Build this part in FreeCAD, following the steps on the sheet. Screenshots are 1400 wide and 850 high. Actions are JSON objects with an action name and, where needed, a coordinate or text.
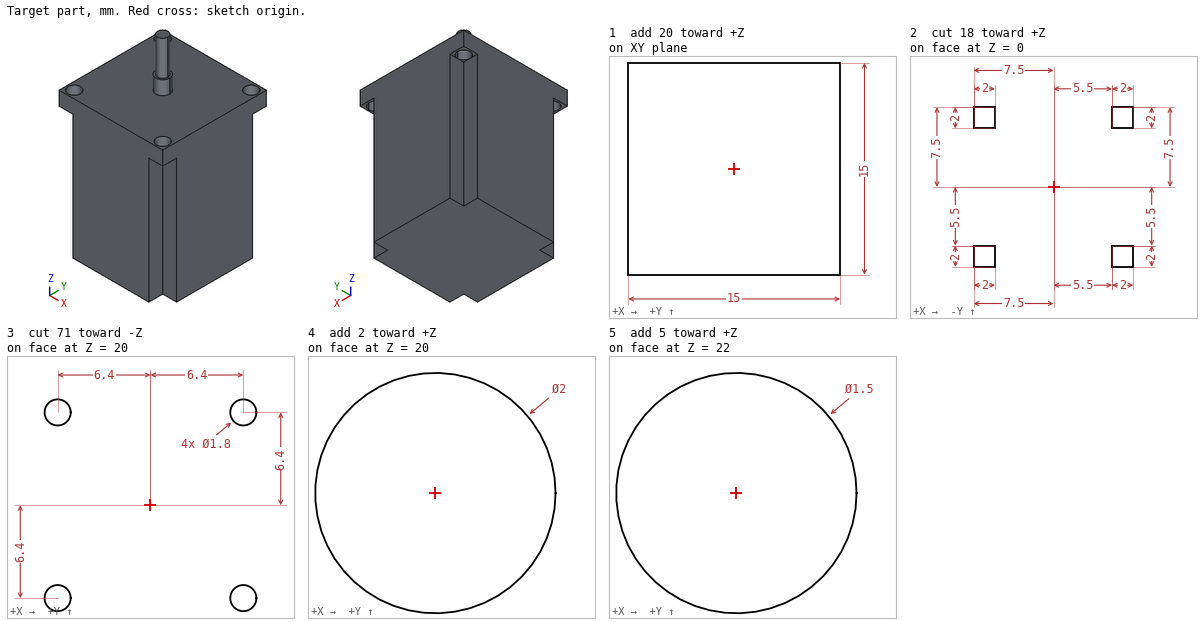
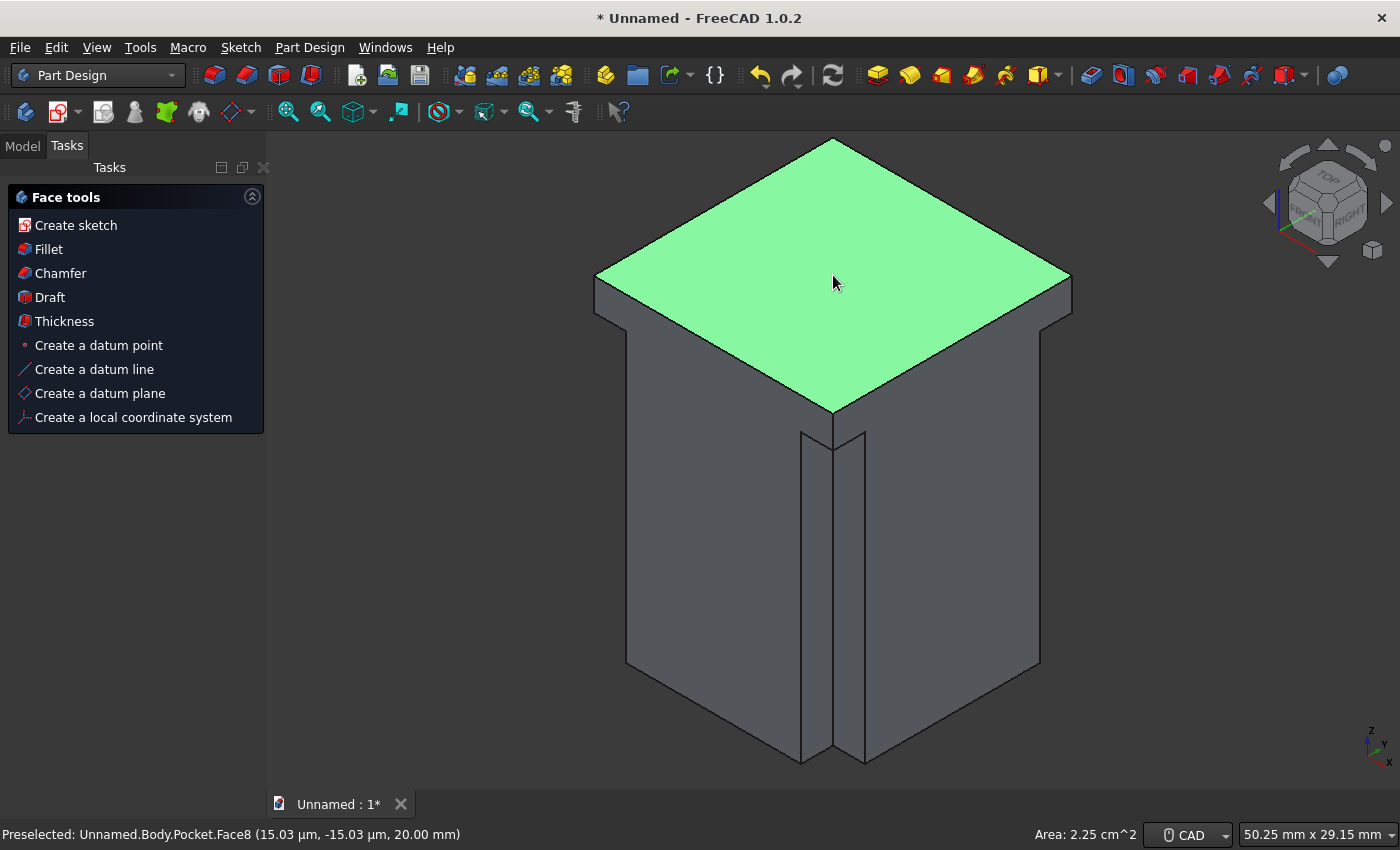
{"action": "left_click", "coordinate": [58, 112]}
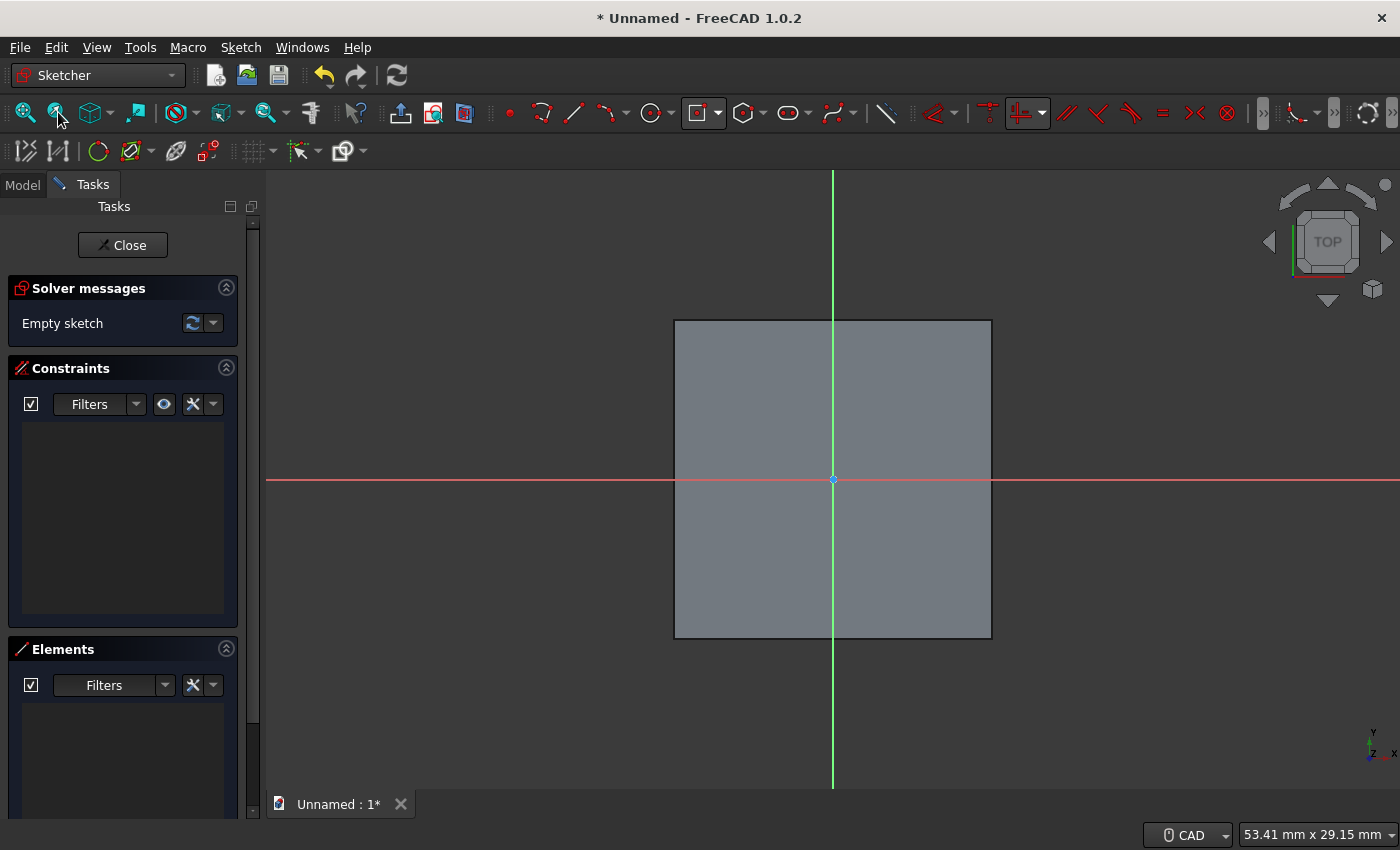
{"action": "left_click", "coordinate": [652, 114]}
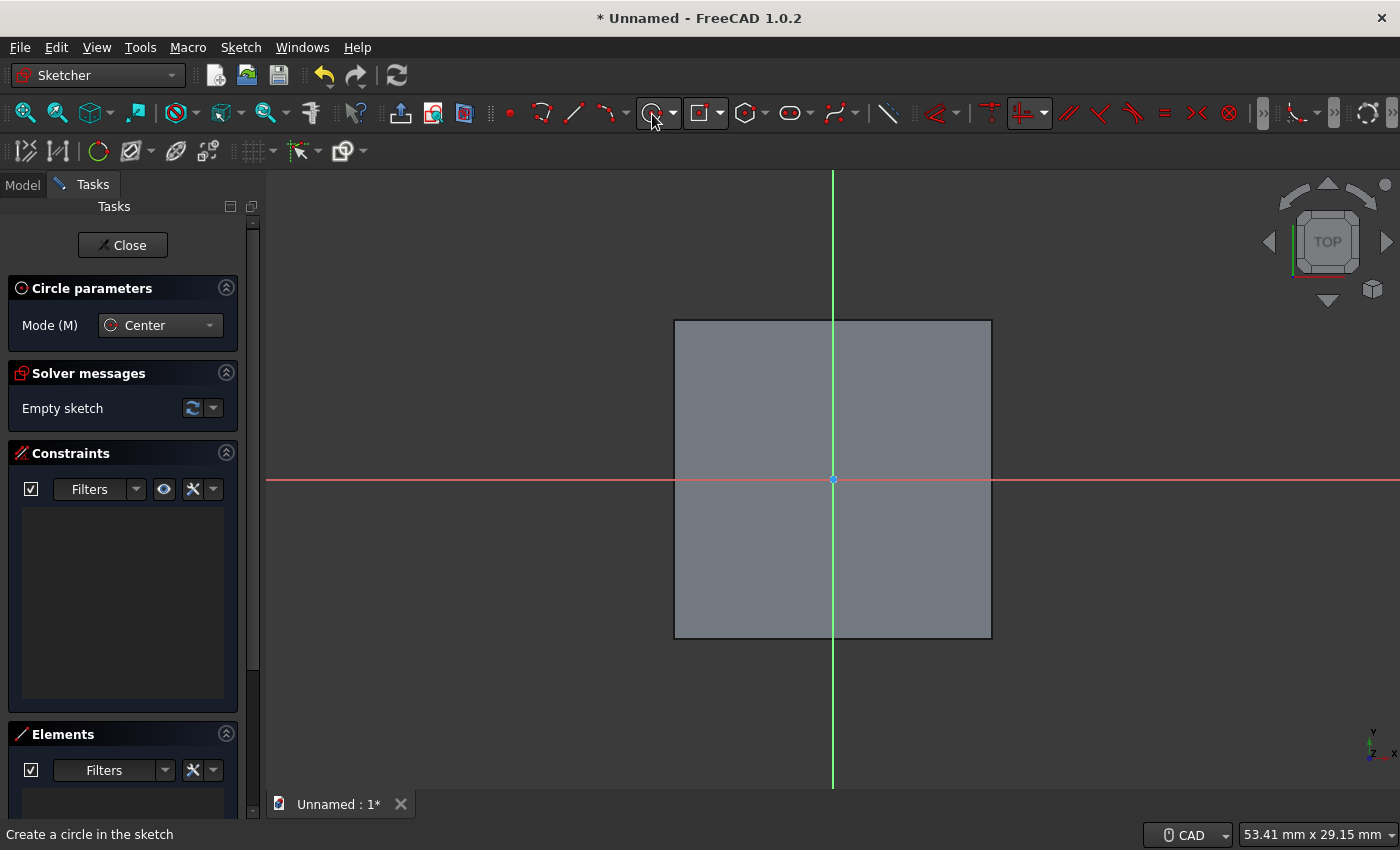
{"action": "left_click", "coordinate": [969, 344]}
{"action": "mouse_move", "coordinate": [982, 330]}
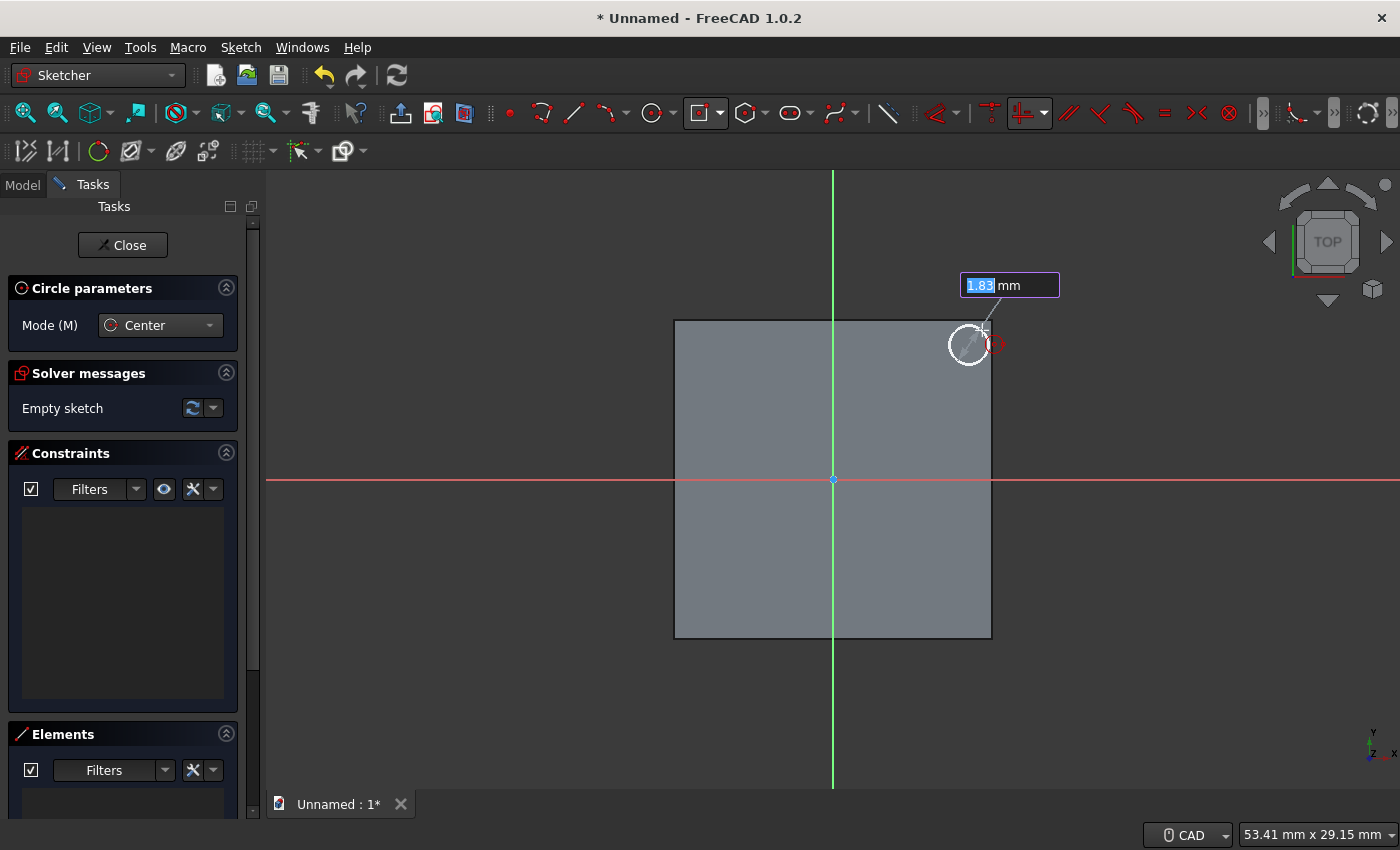
{"action": "type", "text": "1.8"}
{"action": "key", "text": "Return"}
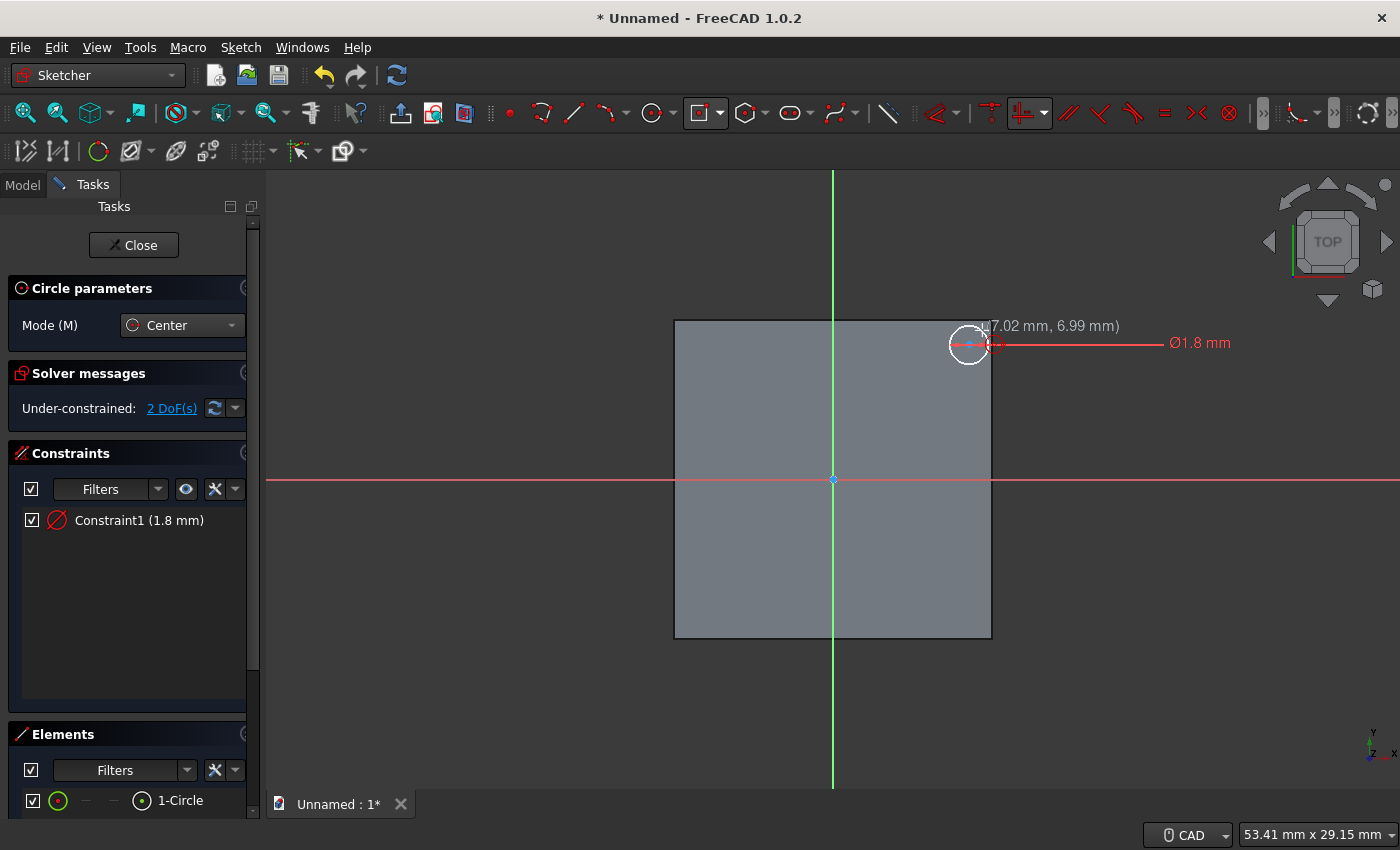
{"action": "left_click", "coordinate": [697, 344]}
{"action": "mouse_move", "coordinate": [711, 330]}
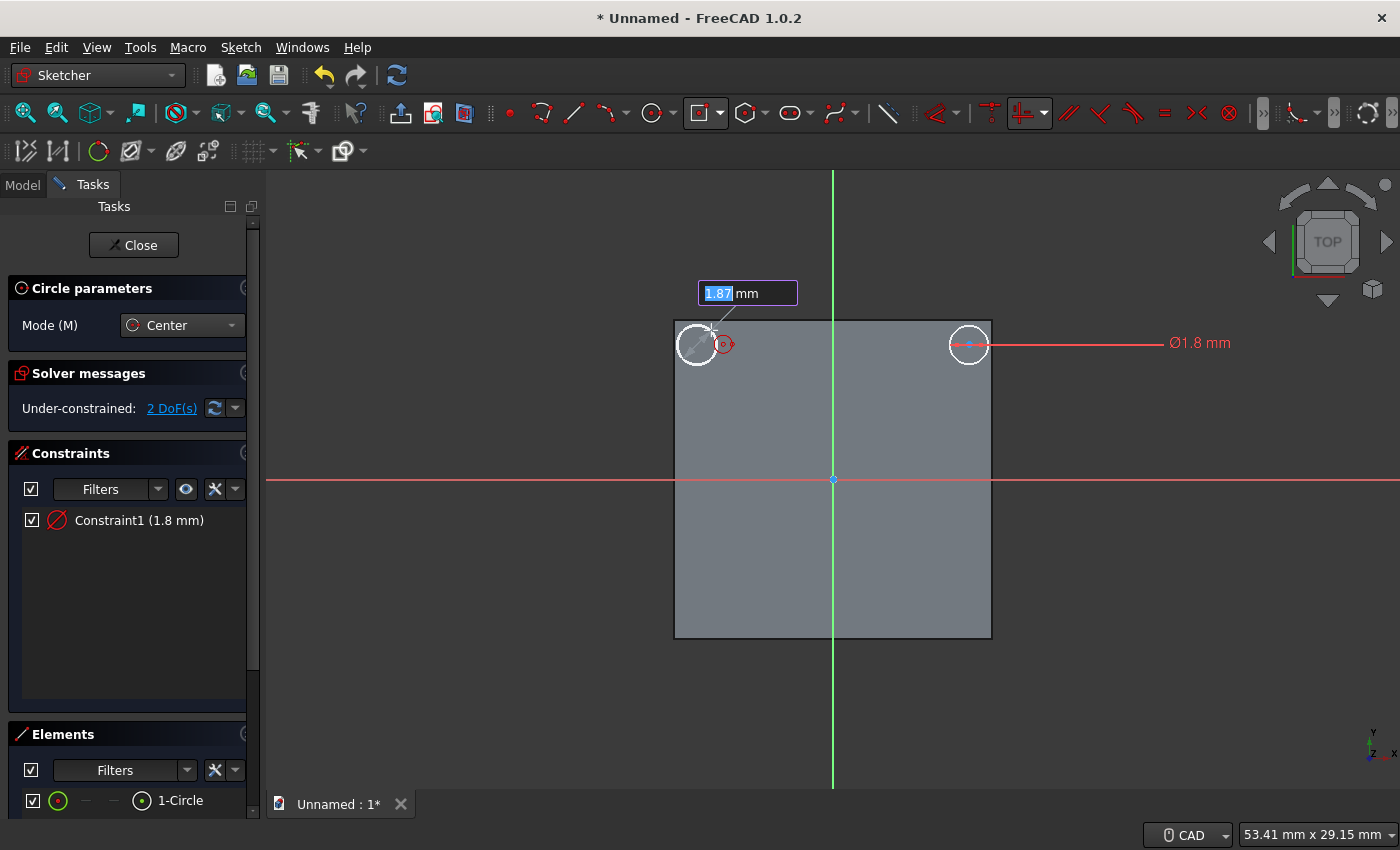
{"action": "type", "text": "1.8"}
{"action": "key", "text": "Return"}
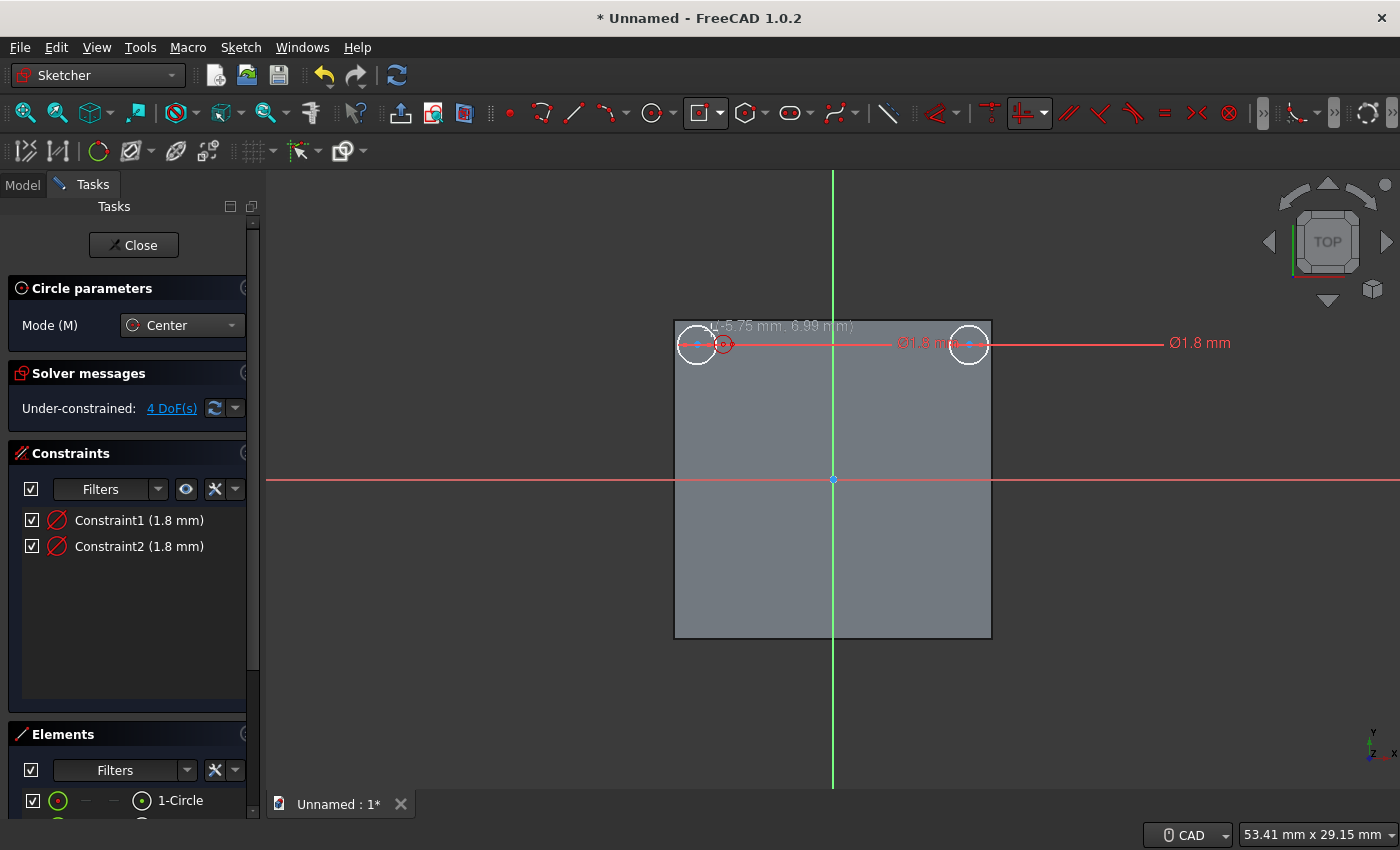
{"action": "left_click", "coordinate": [697, 615]}
{"action": "mouse_move", "coordinate": [711, 602]}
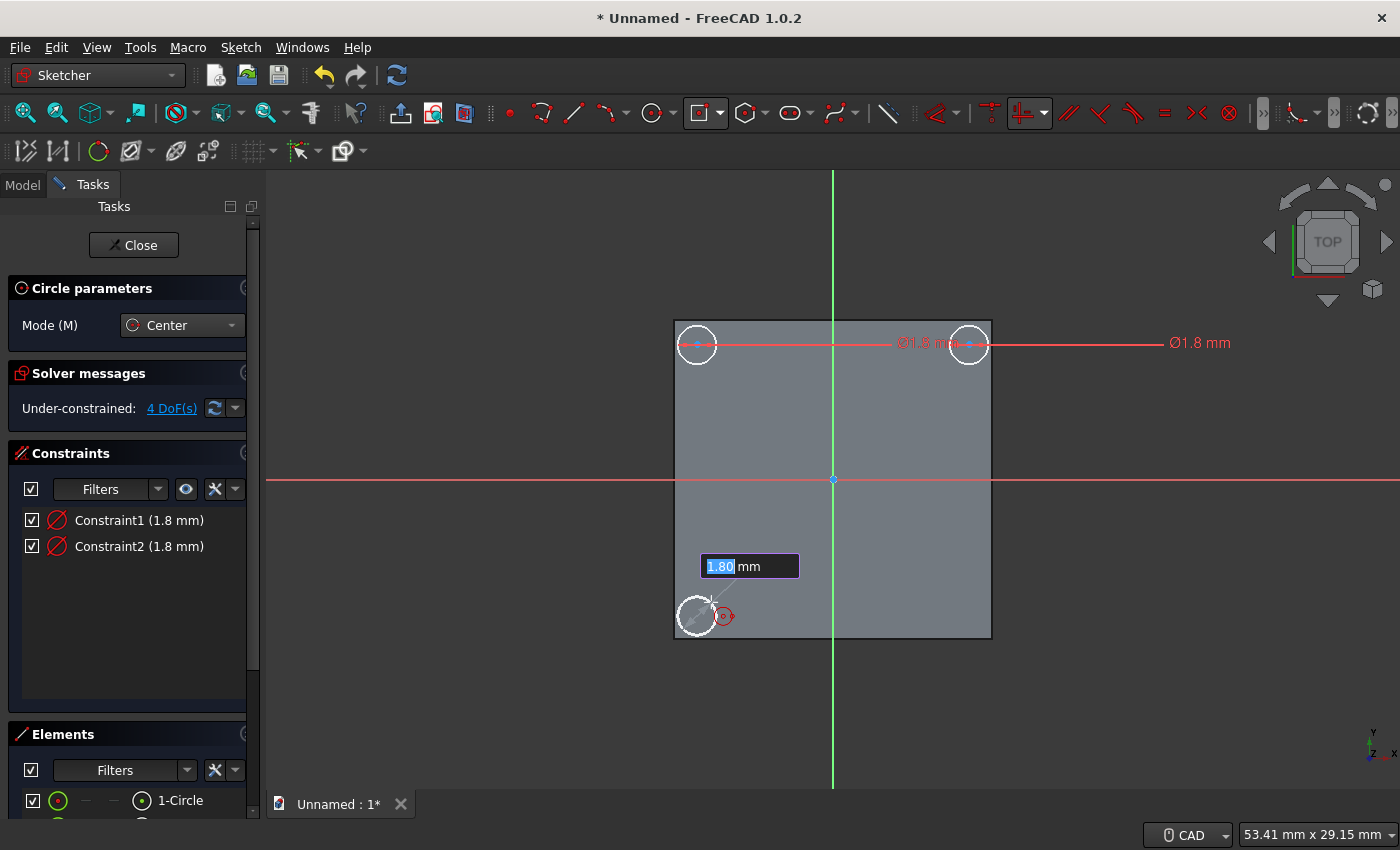
{"action": "type", "text": "1.8"}
{"action": "key", "text": "Return"}